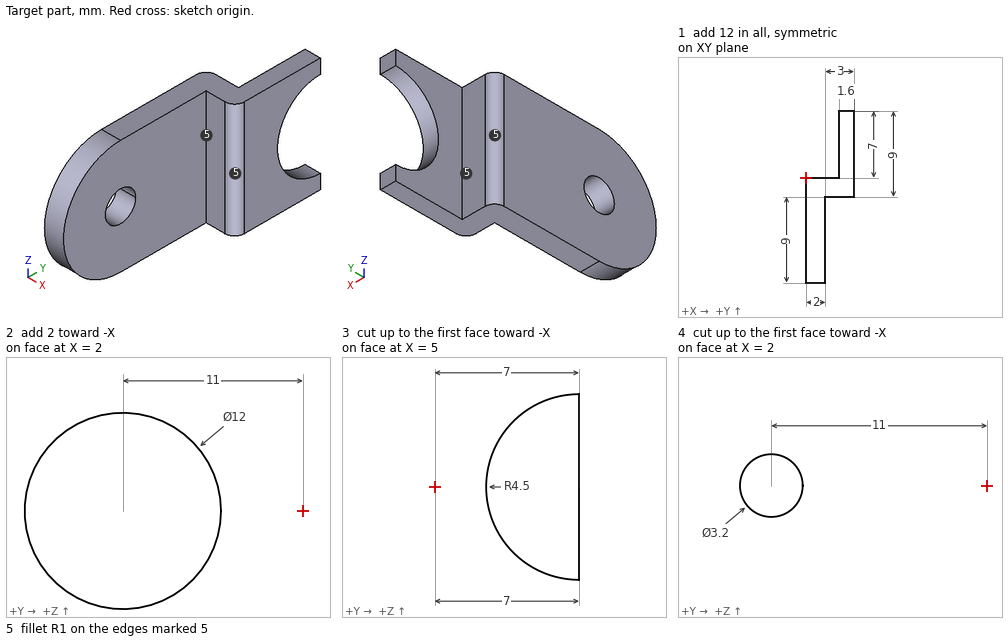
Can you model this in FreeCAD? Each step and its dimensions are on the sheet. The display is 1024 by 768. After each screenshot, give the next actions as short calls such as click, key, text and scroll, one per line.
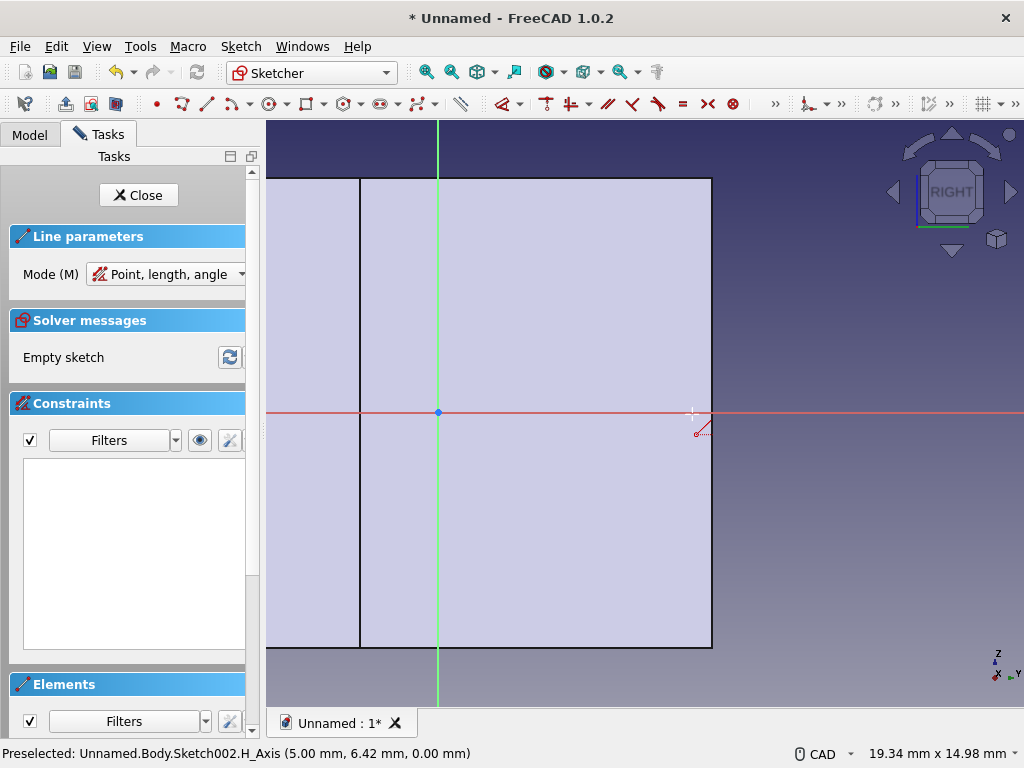
click(712, 589)
click(712, 236)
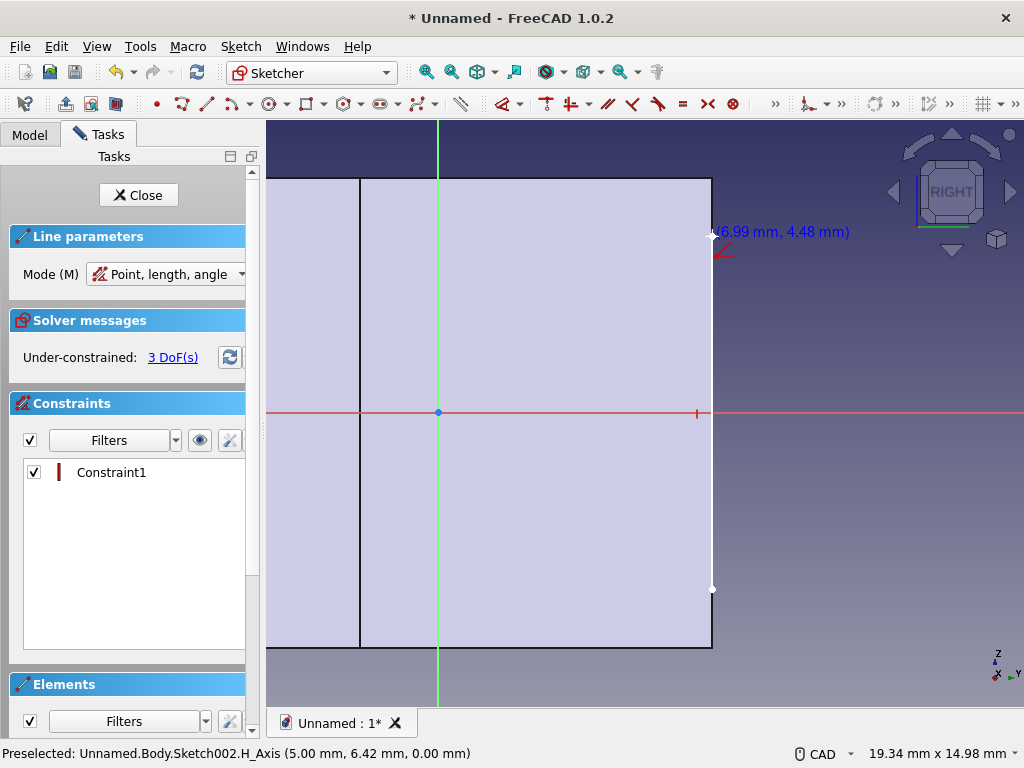
key(g)
key(3)
key(a)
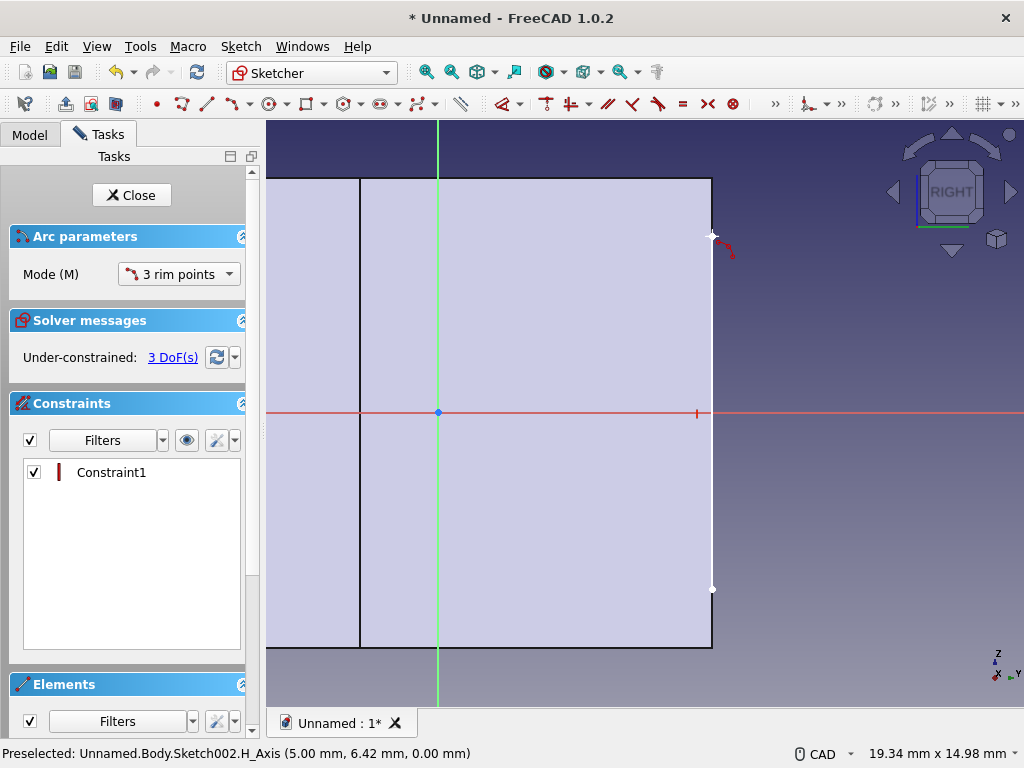
click(712, 237)
click(712, 590)
click(545, 358)
key(Escape)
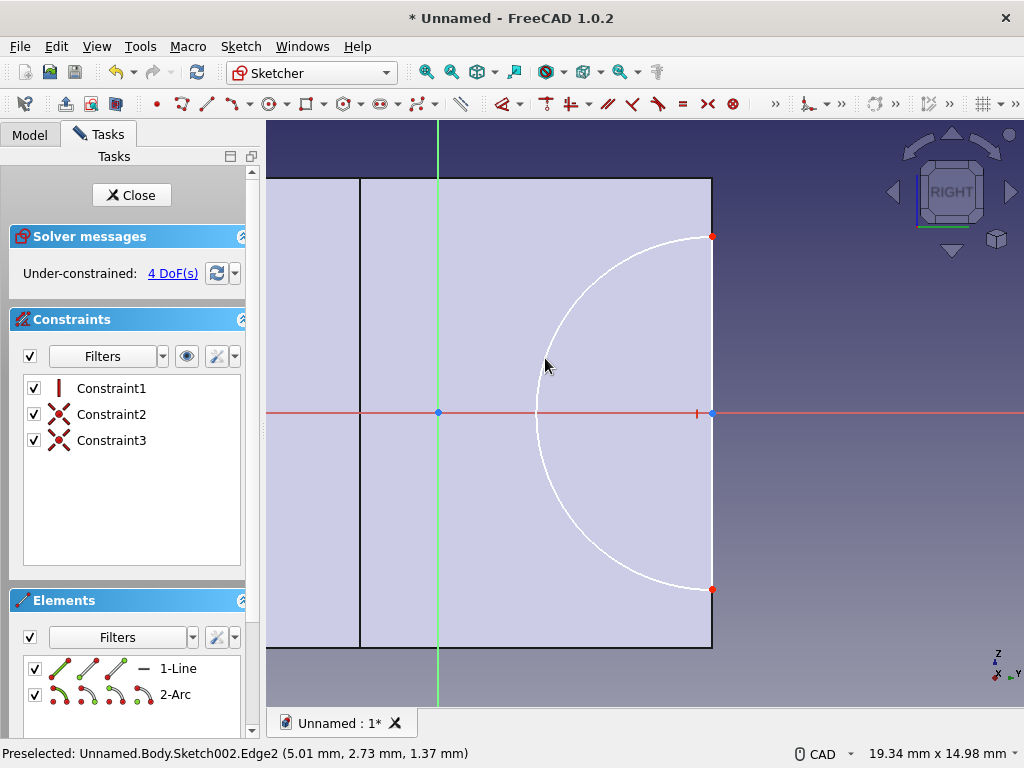
click(713, 413)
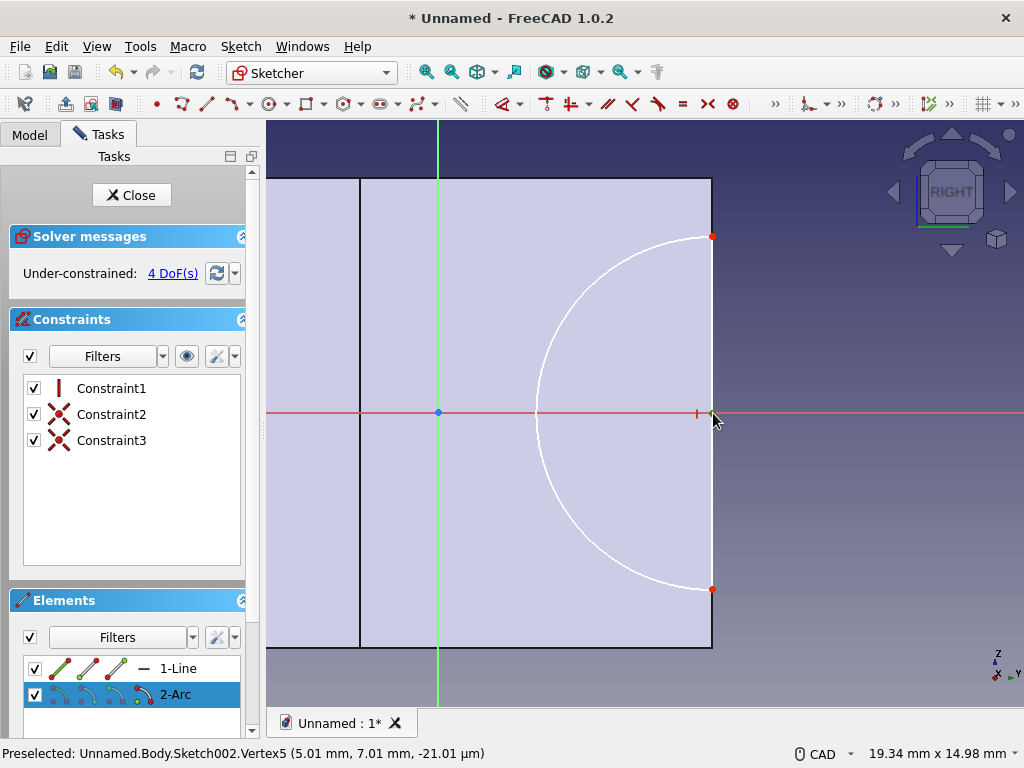
click(334, 413)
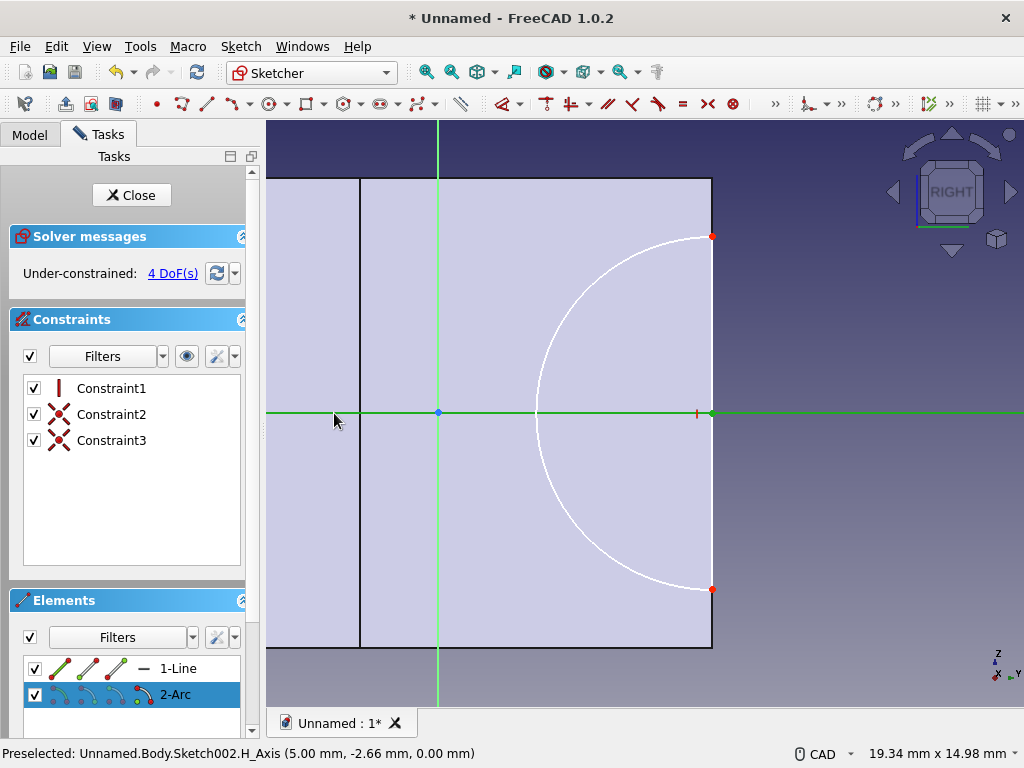
key(c)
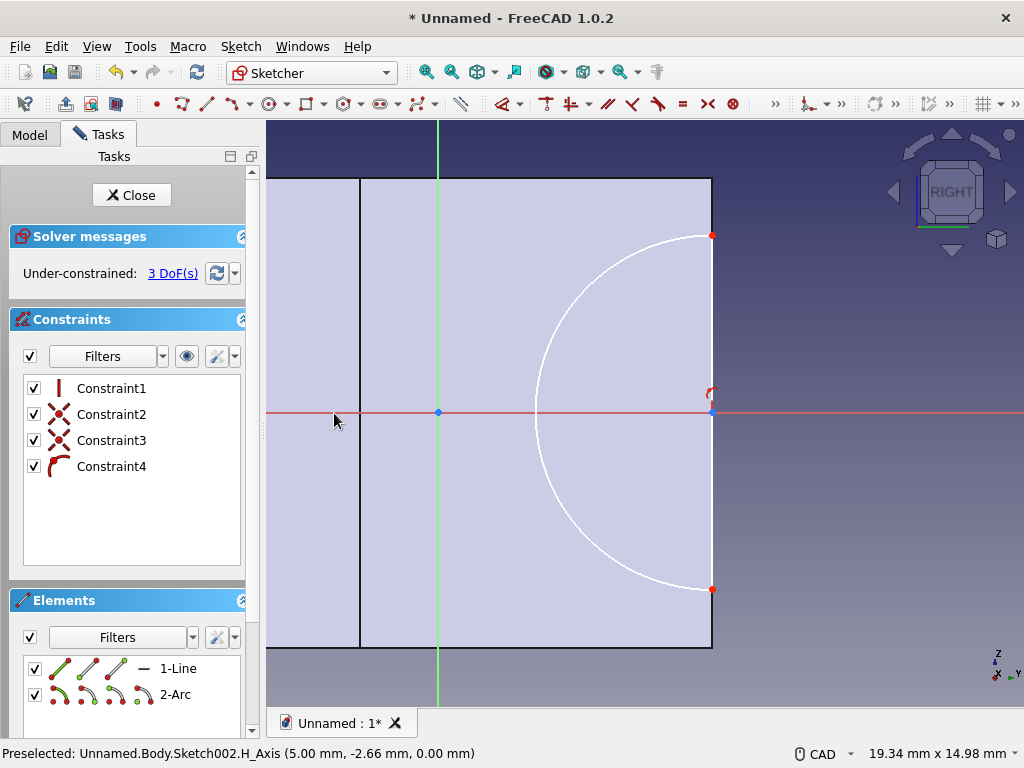
key(d)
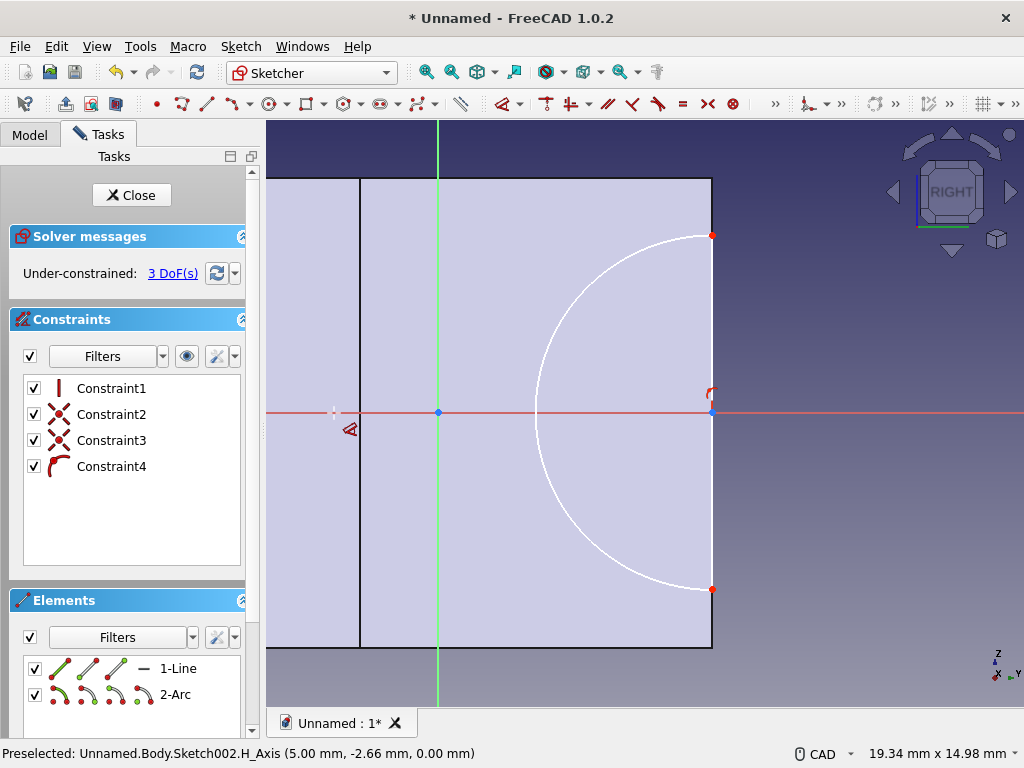
click(569, 309)
click(543, 290)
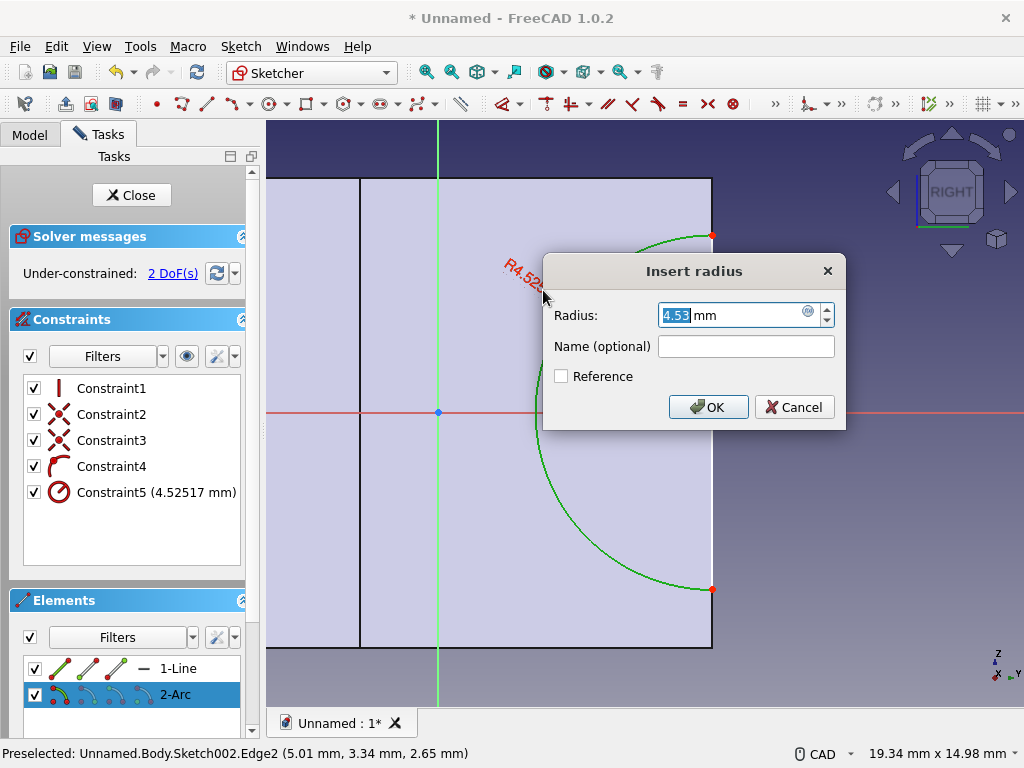
text(4.5)
key(Return)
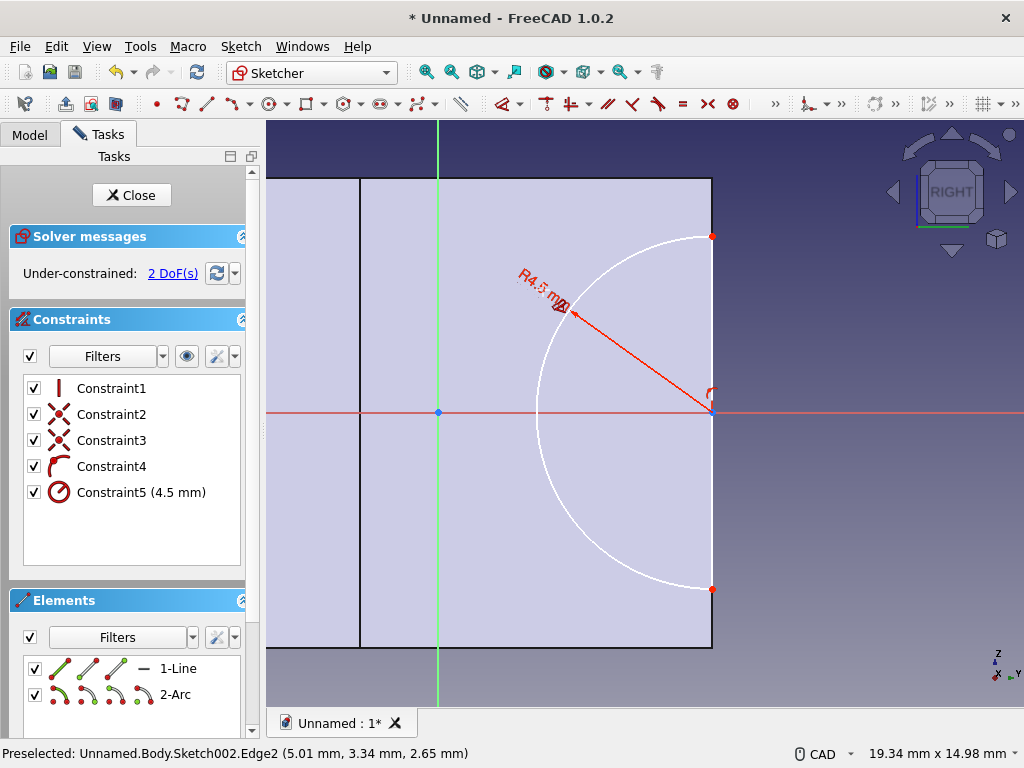
click(712, 589)
click(575, 623)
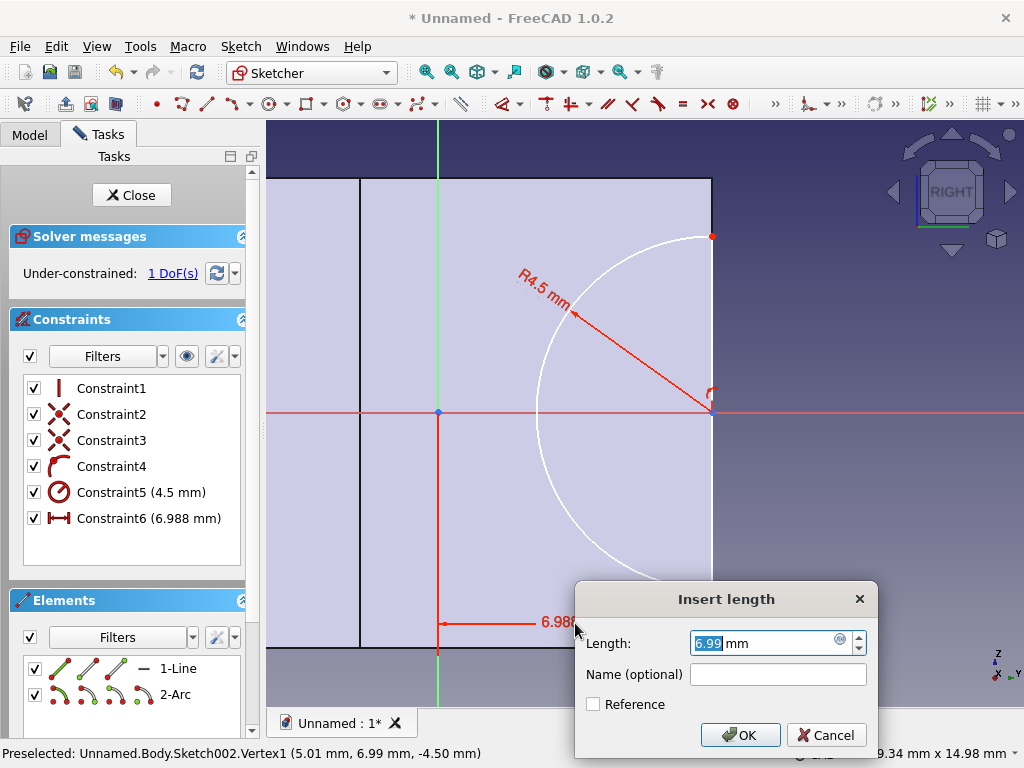
text(7)
key(Return)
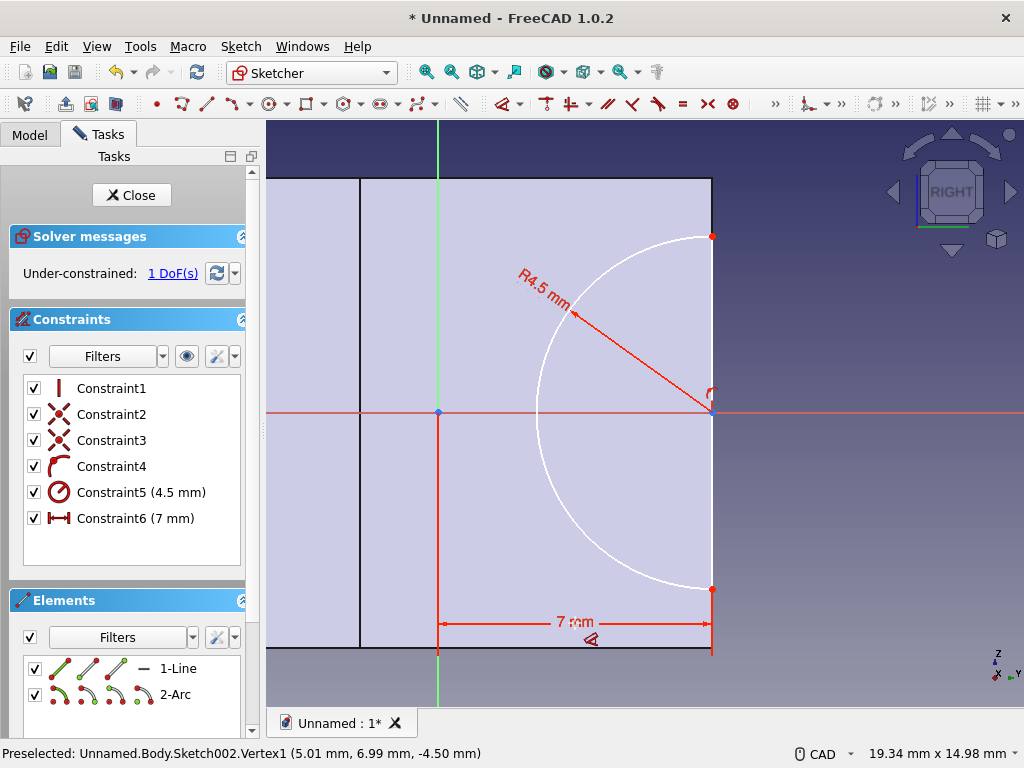
click(713, 413)
click(576, 447)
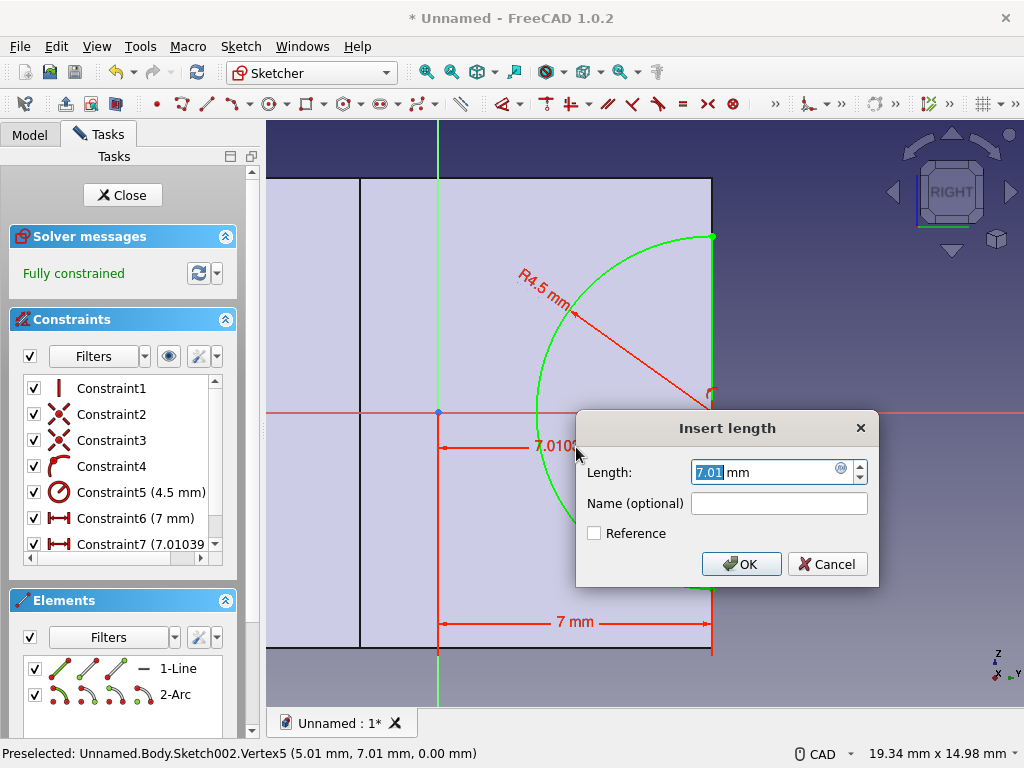
text(7)
key(Return)
key(Escape)